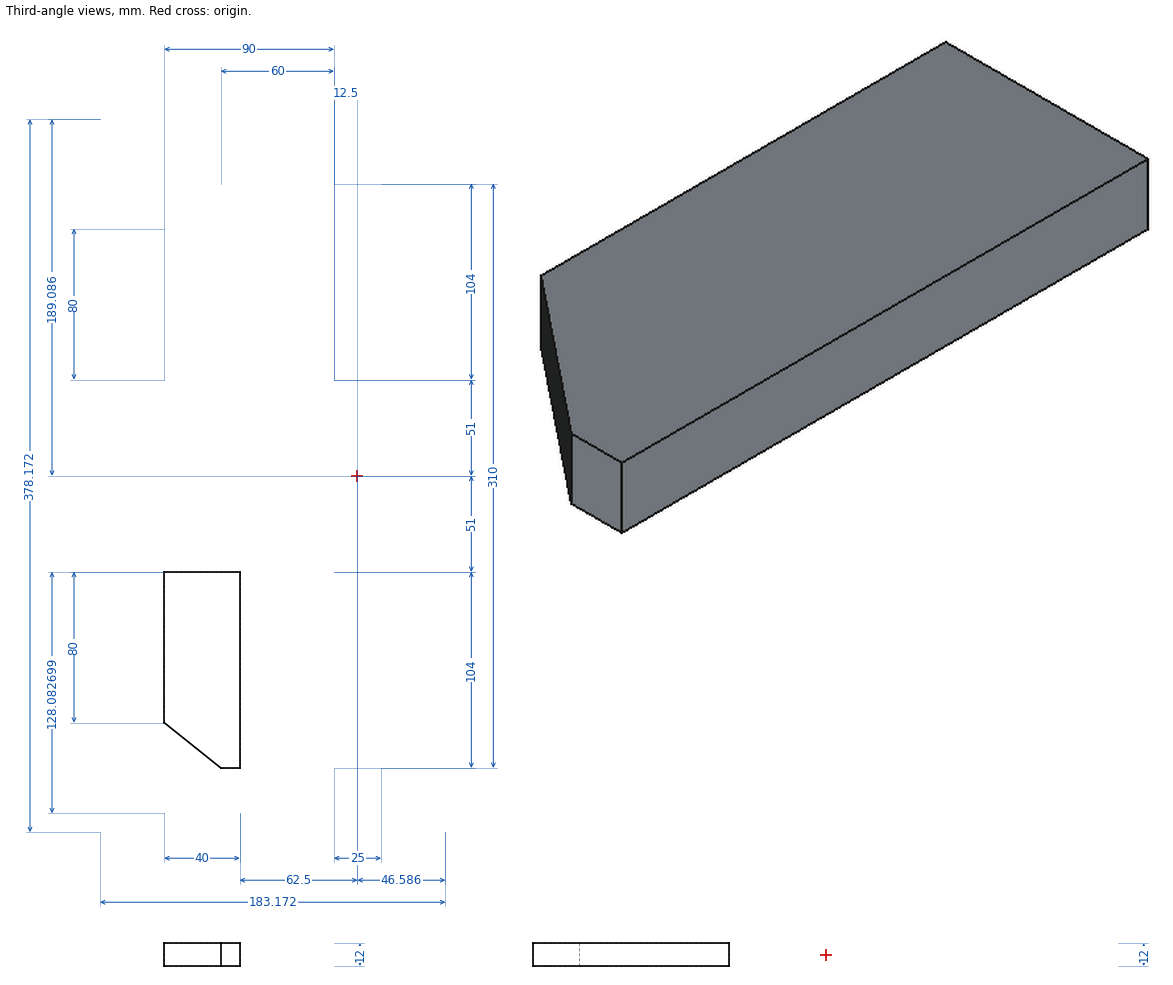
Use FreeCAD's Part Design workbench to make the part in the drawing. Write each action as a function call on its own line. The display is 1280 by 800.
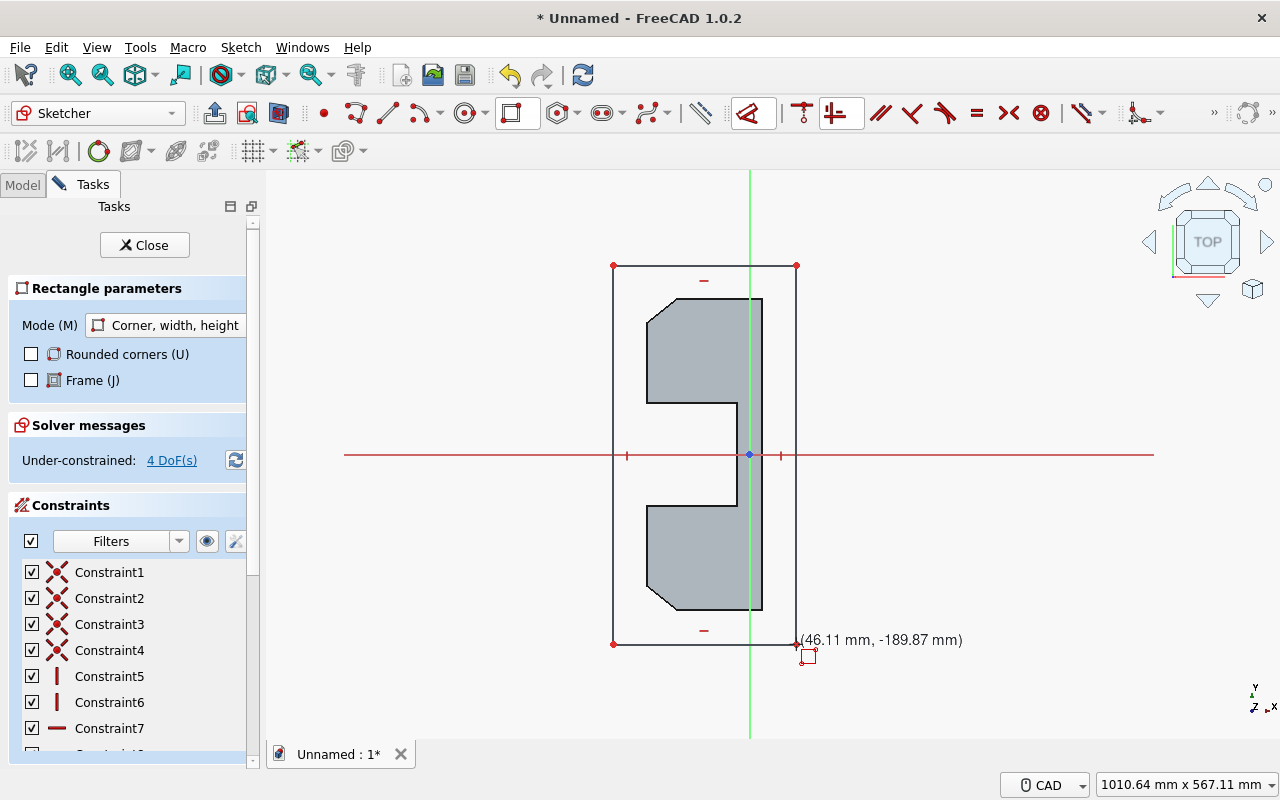
click(647, 506)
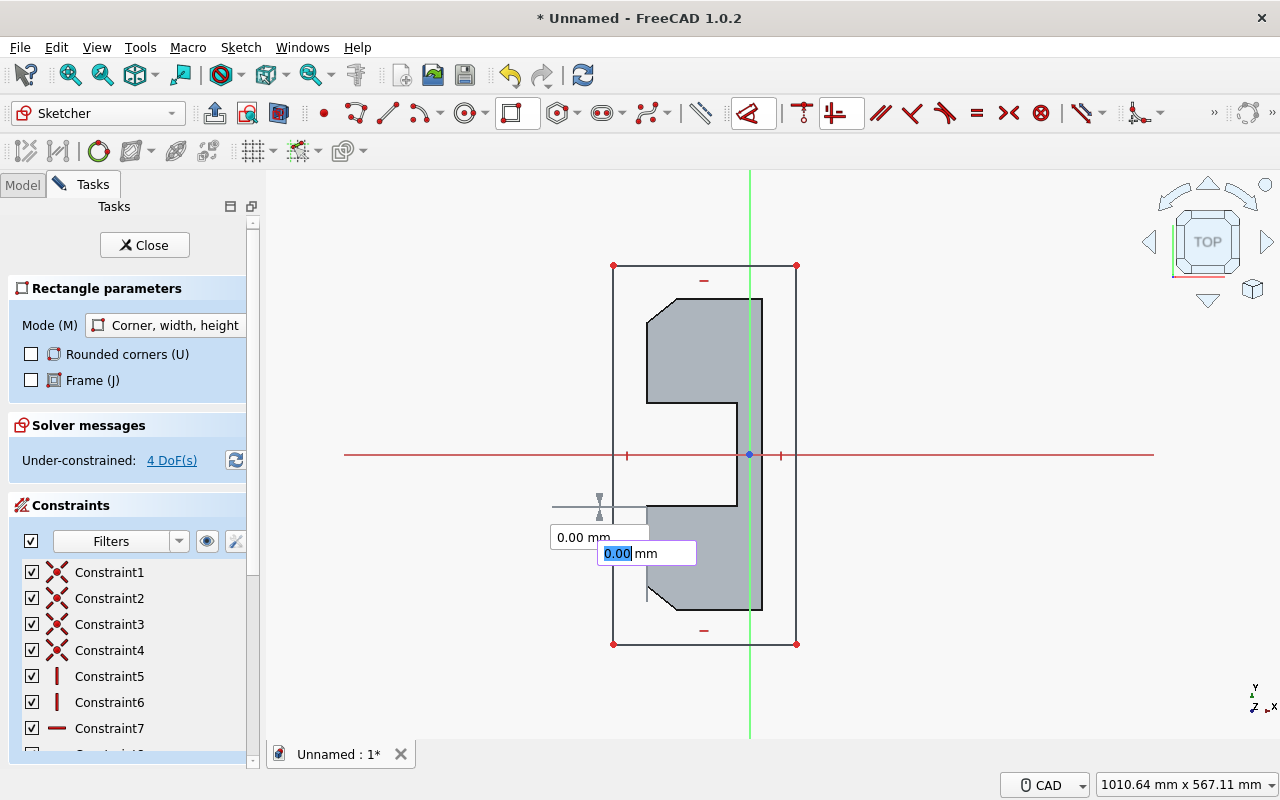
scroll(687, 634, up, 3)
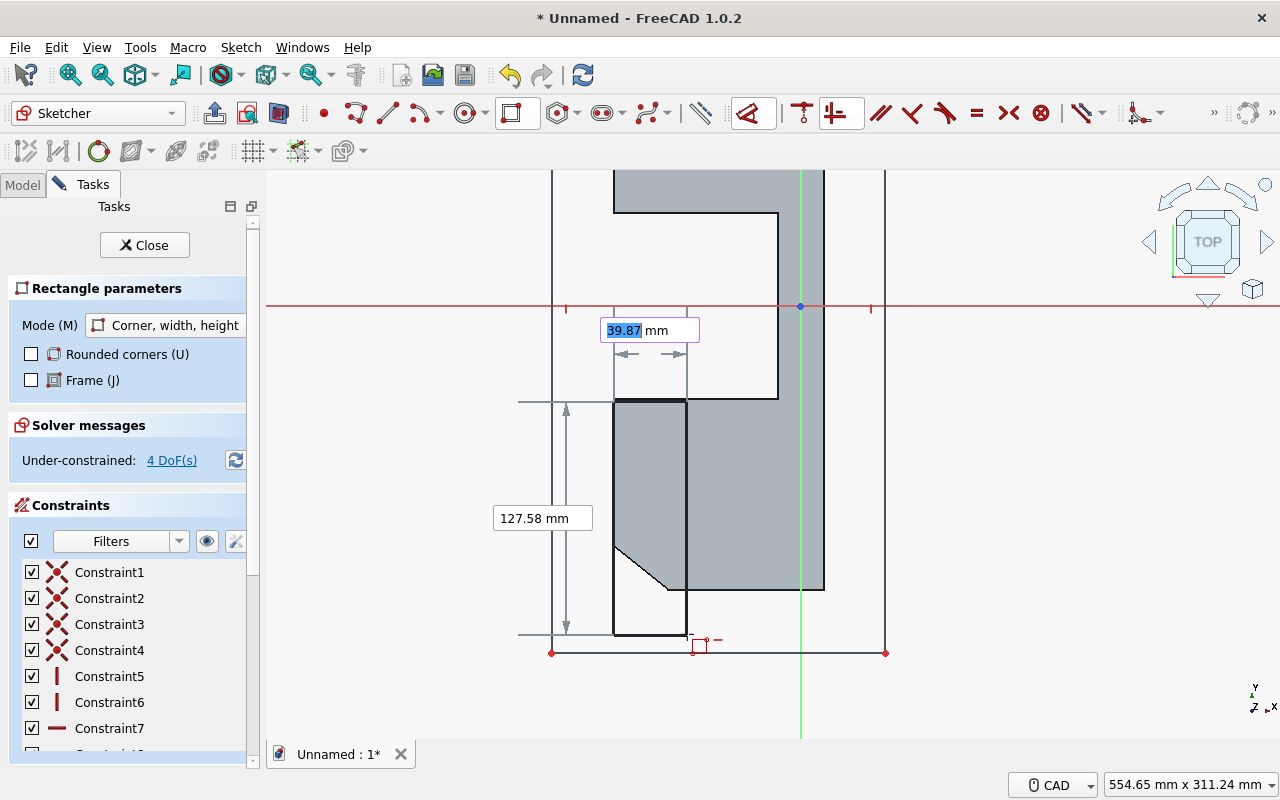
click(687, 634)
key(Escape)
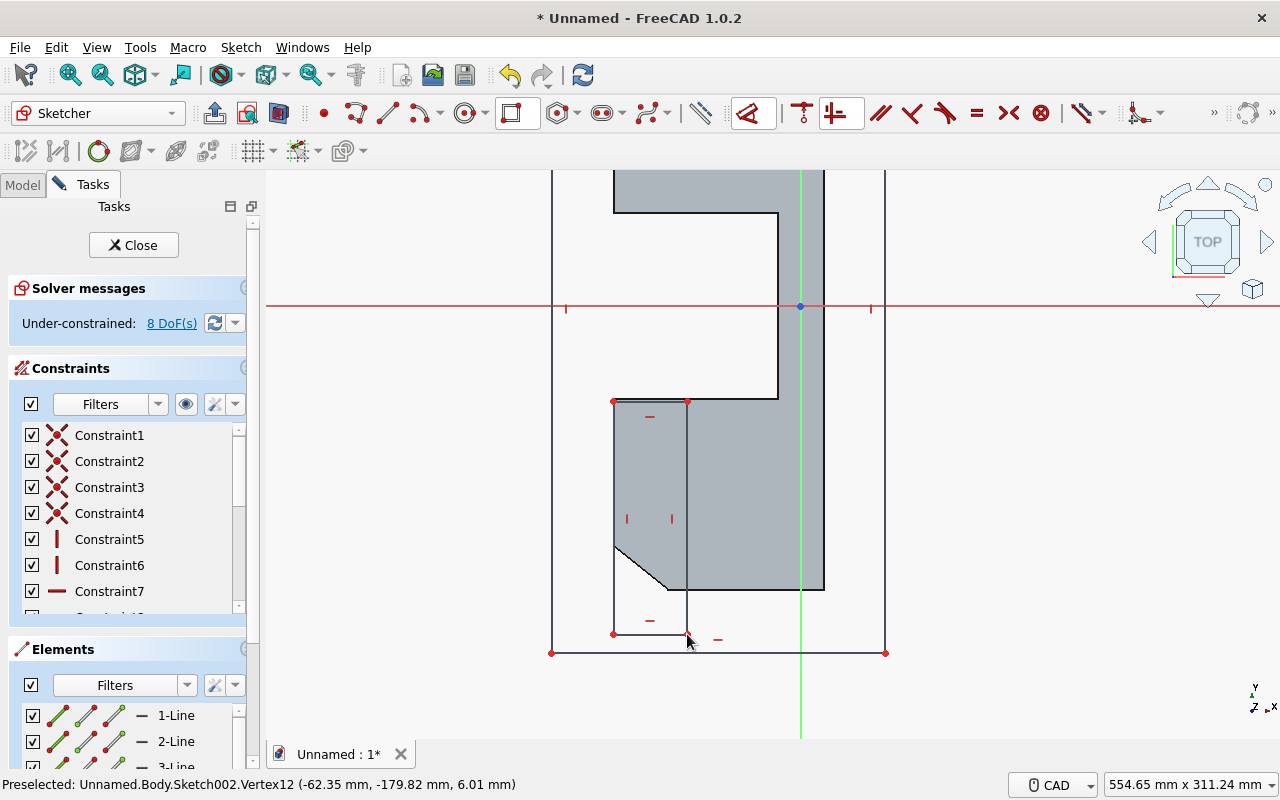
click(636, 635)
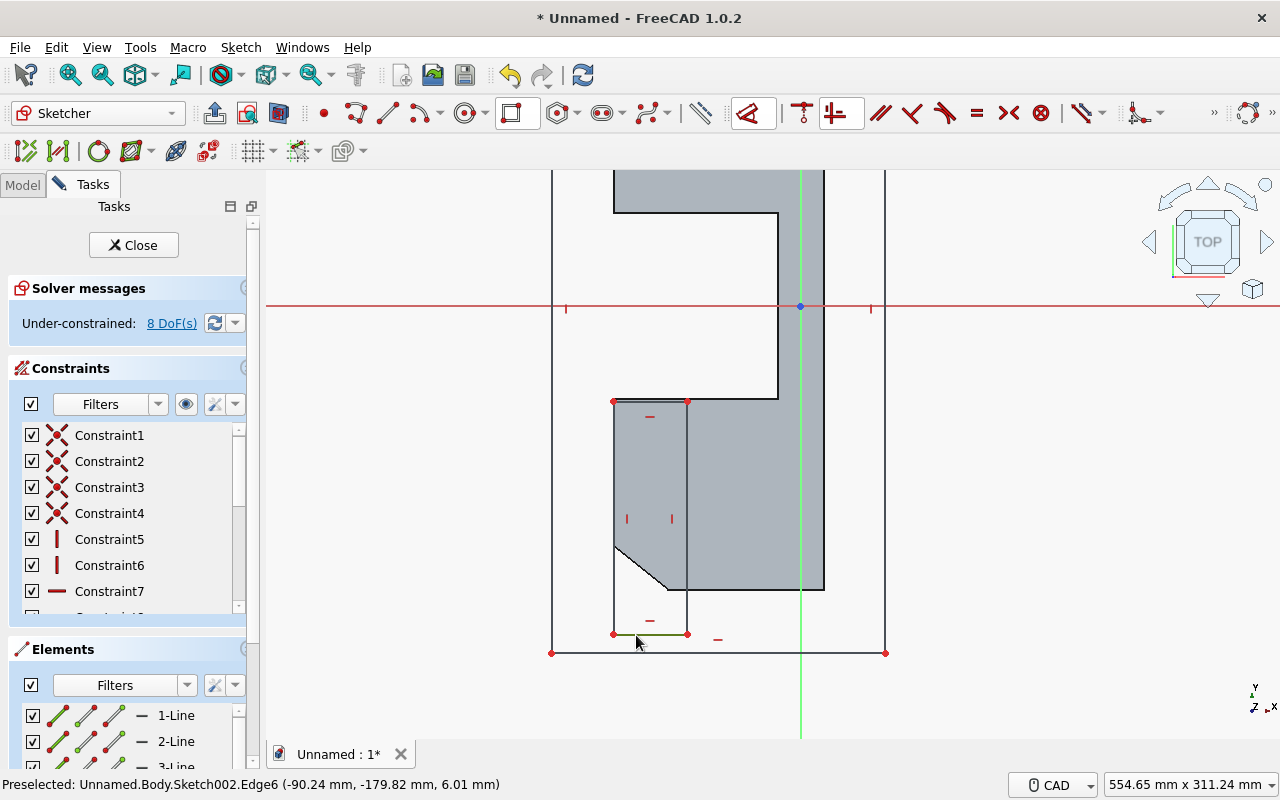
click(770, 114)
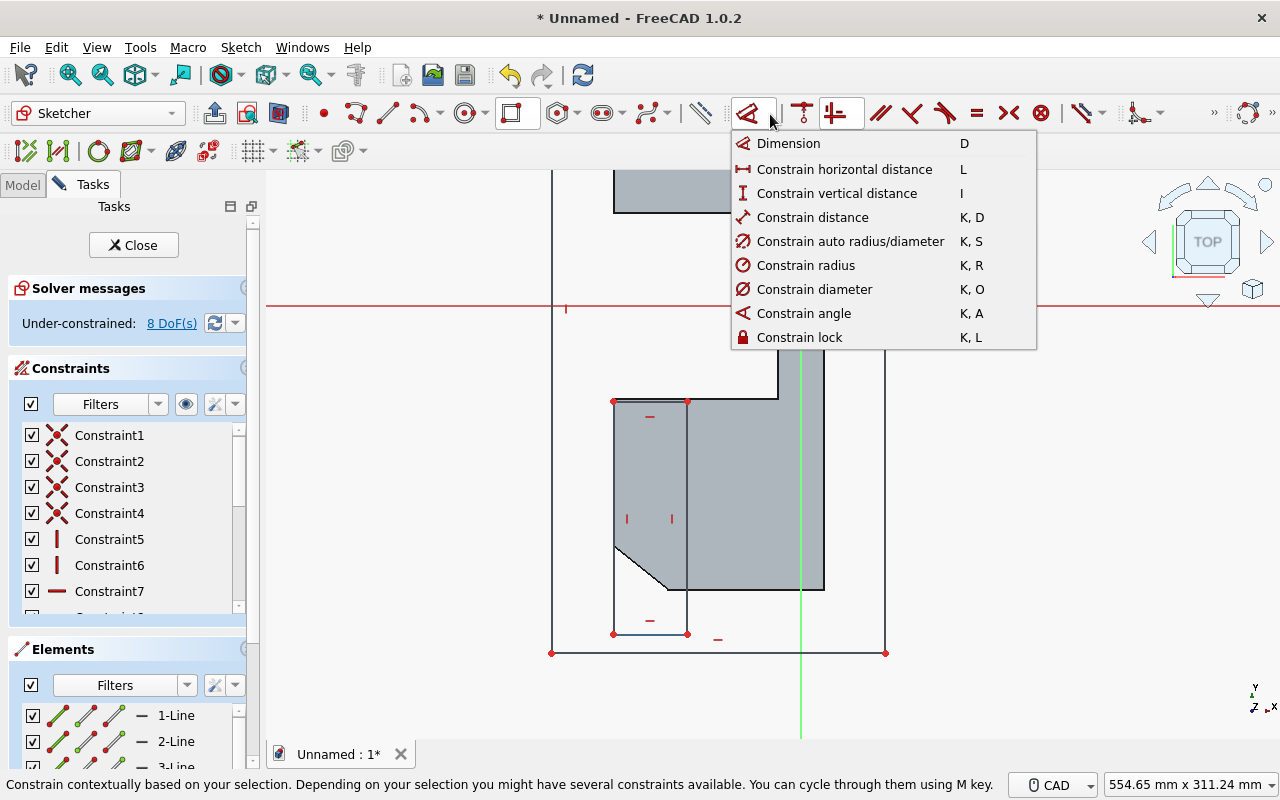
click(884, 169)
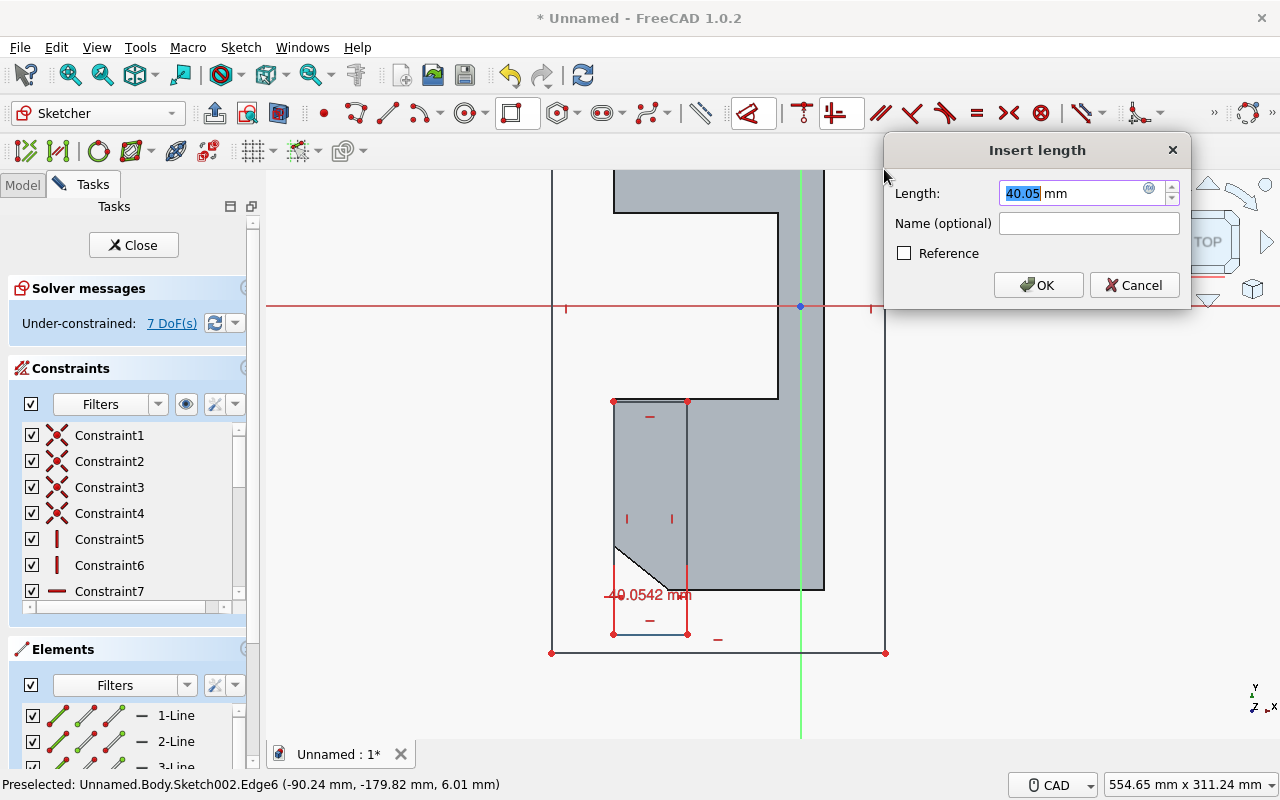
text(40)
key(Return)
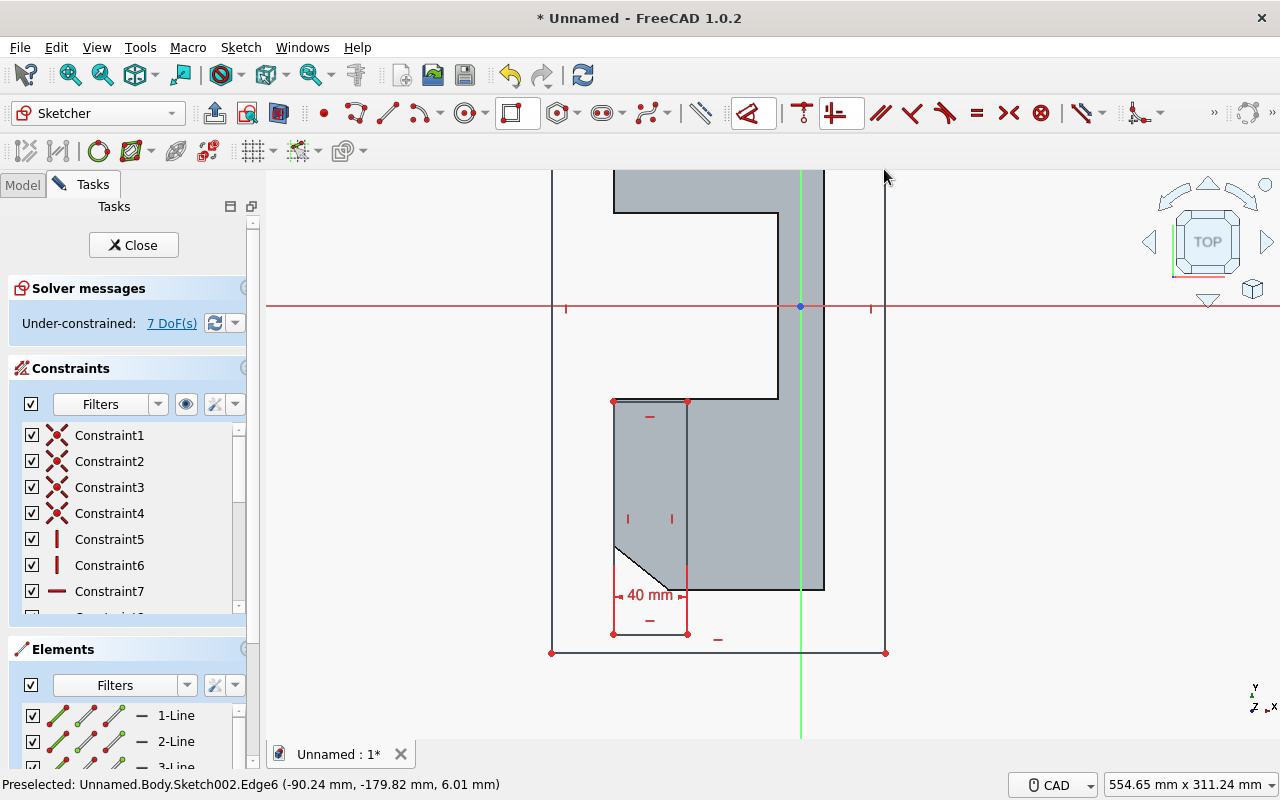
click(614, 402)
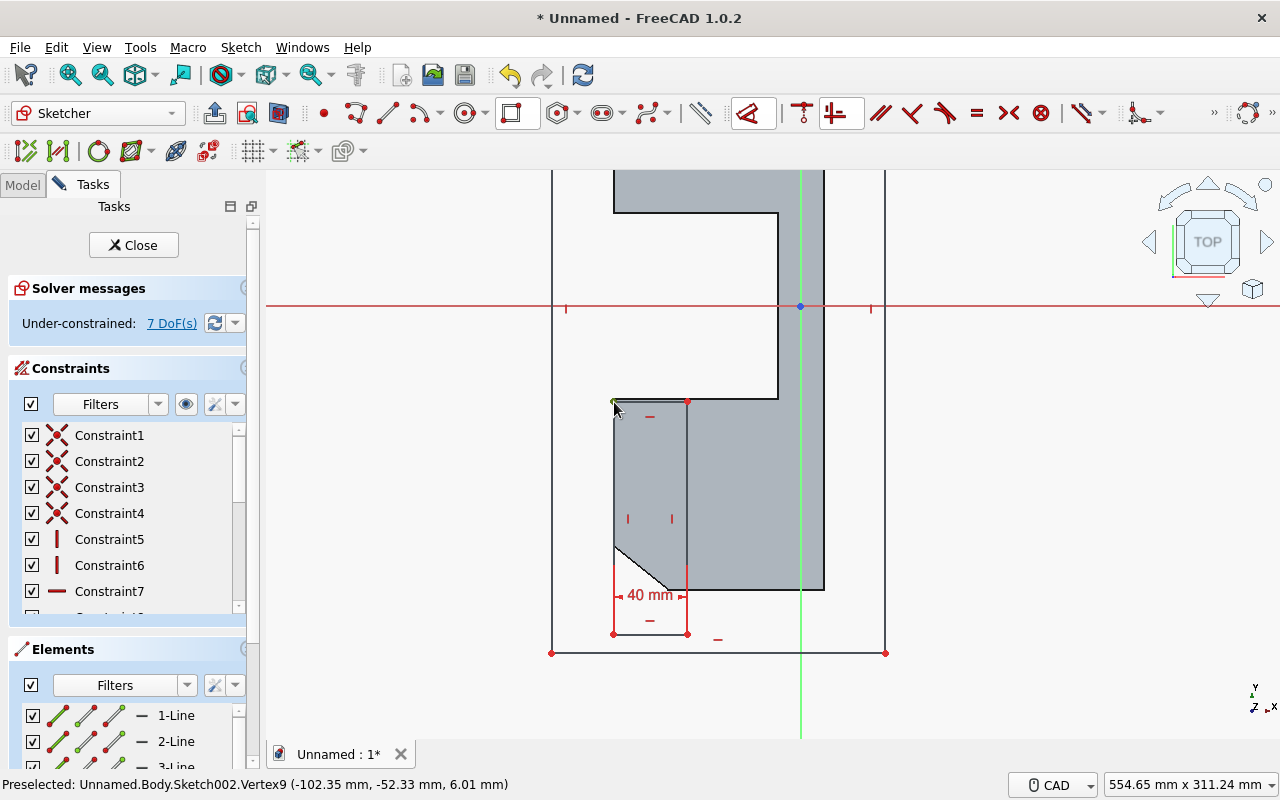
click(770, 114)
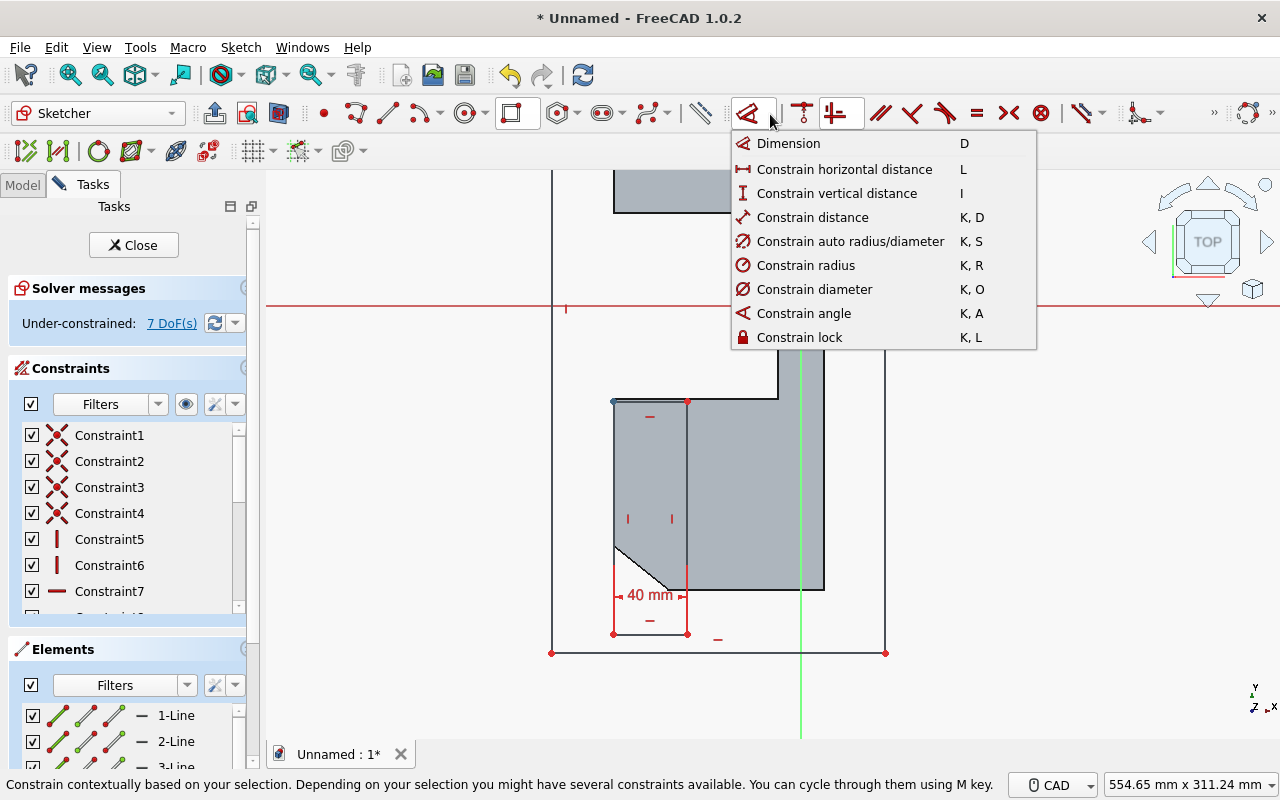
click(884, 193)